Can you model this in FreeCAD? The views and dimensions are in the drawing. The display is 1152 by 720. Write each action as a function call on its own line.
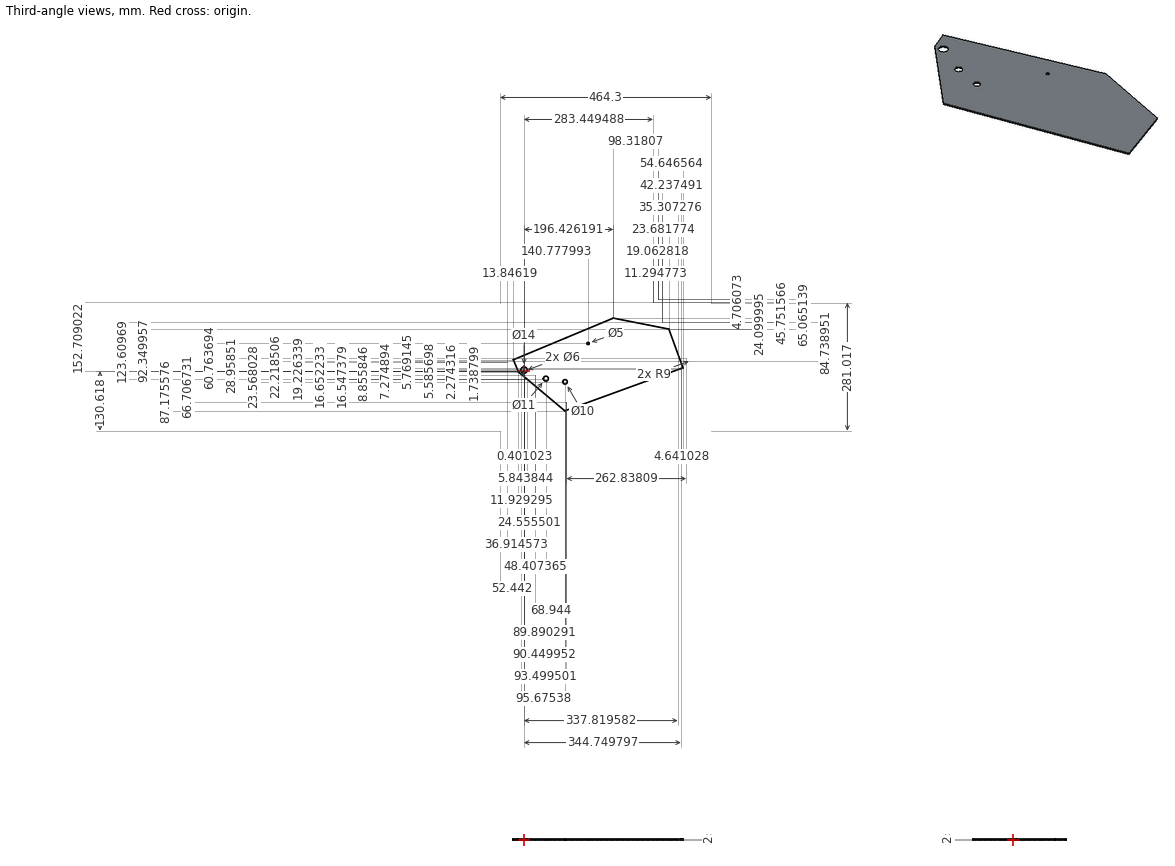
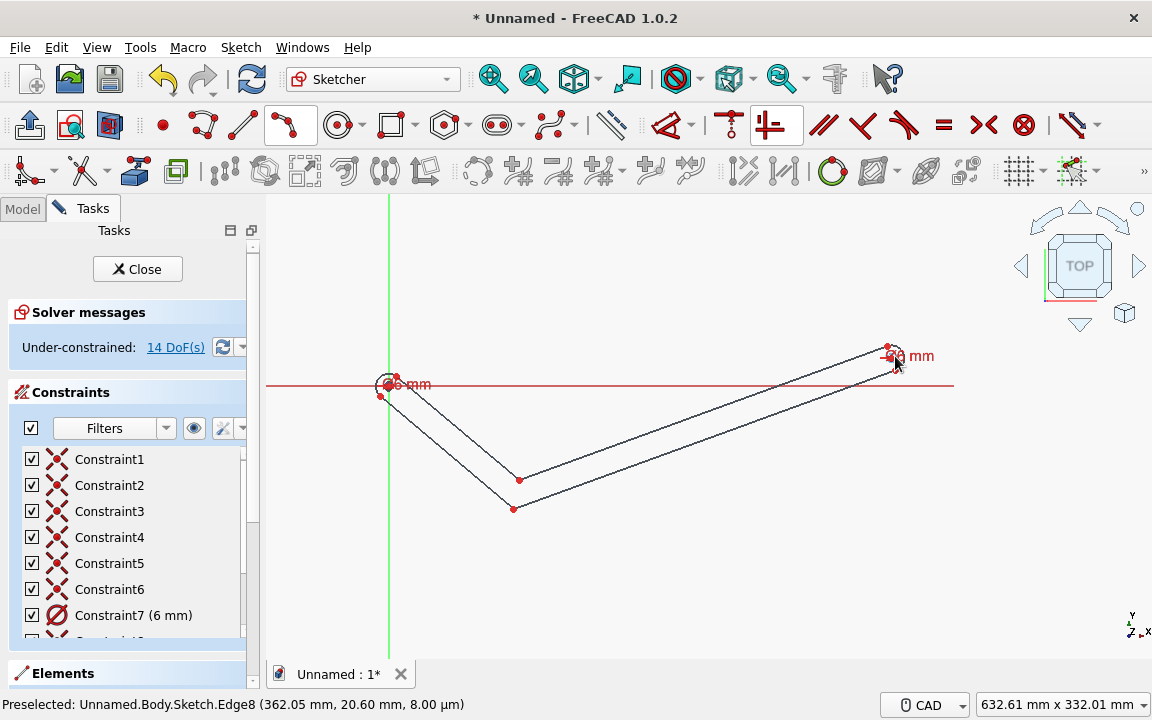
click(777, 386)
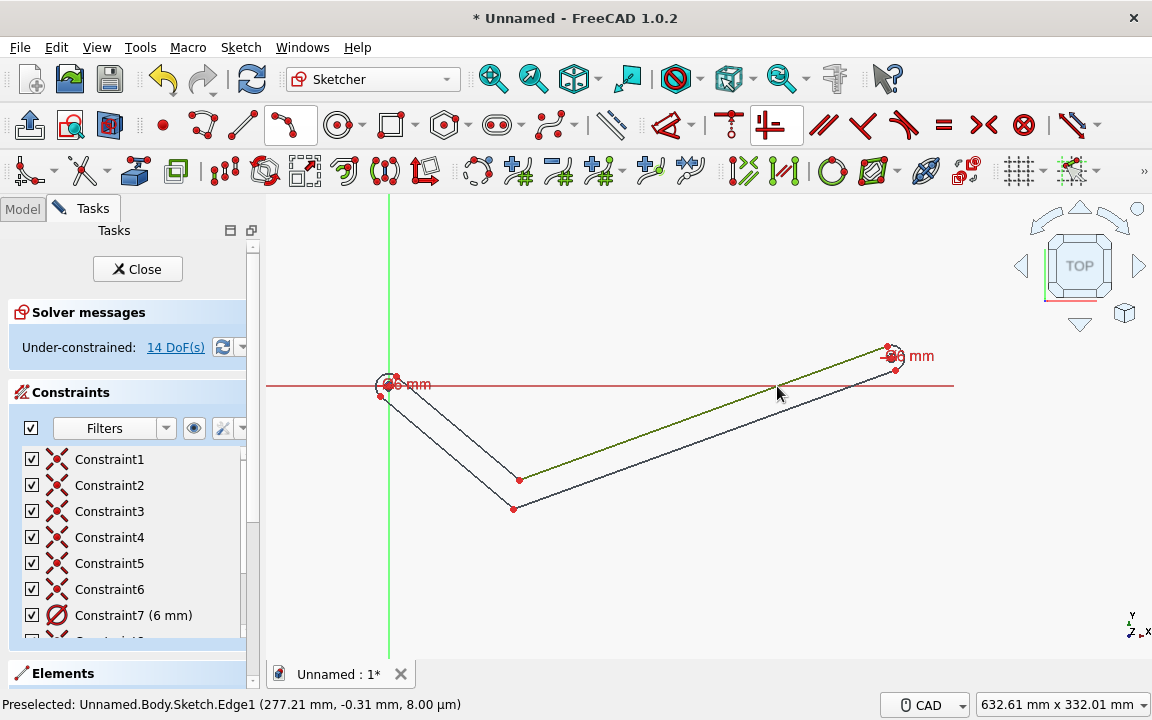
scroll(904, 354, up, 3)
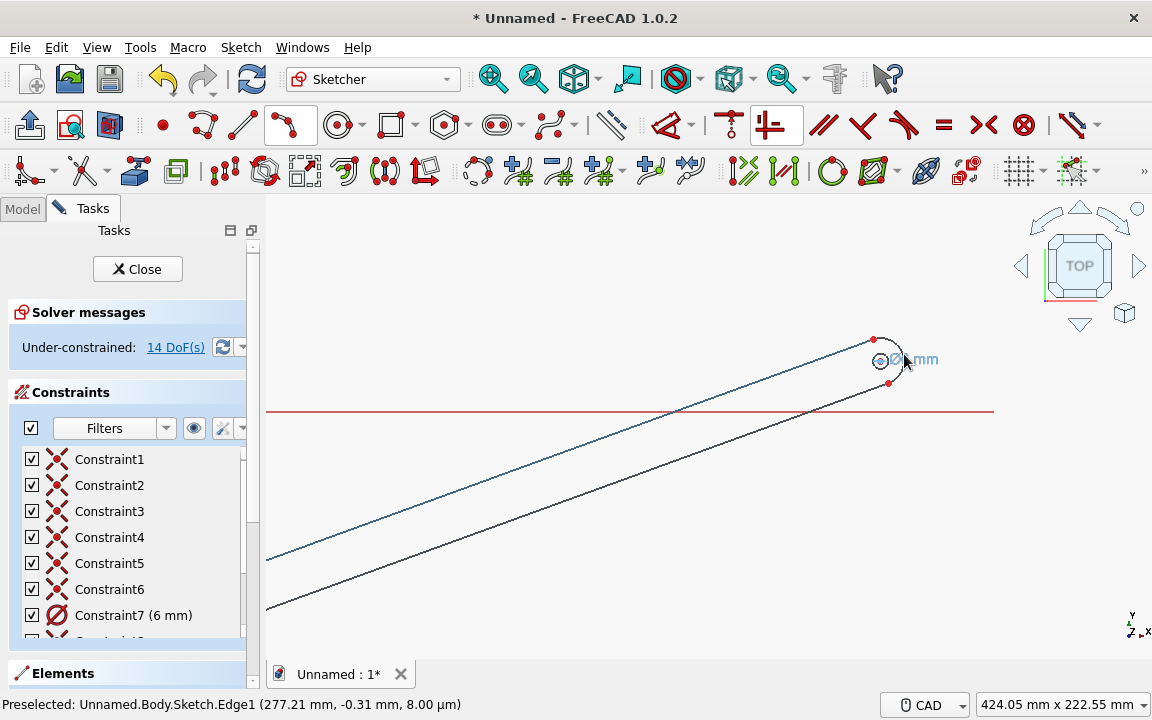
click(894, 342)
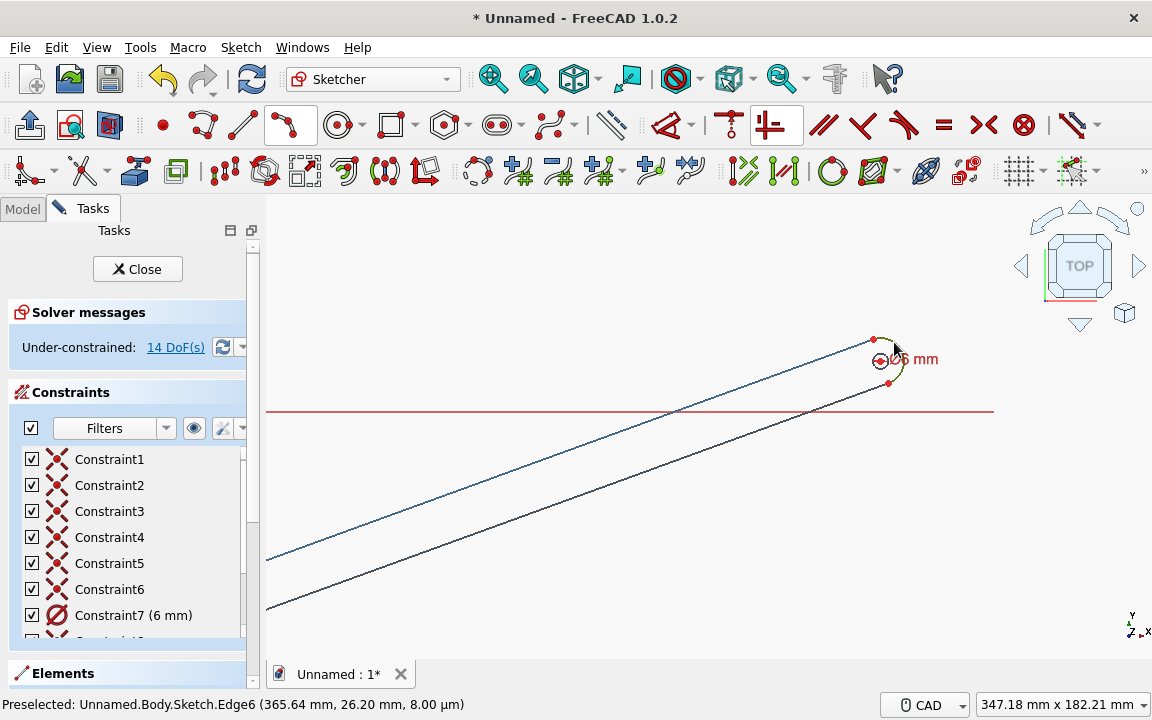
key(t)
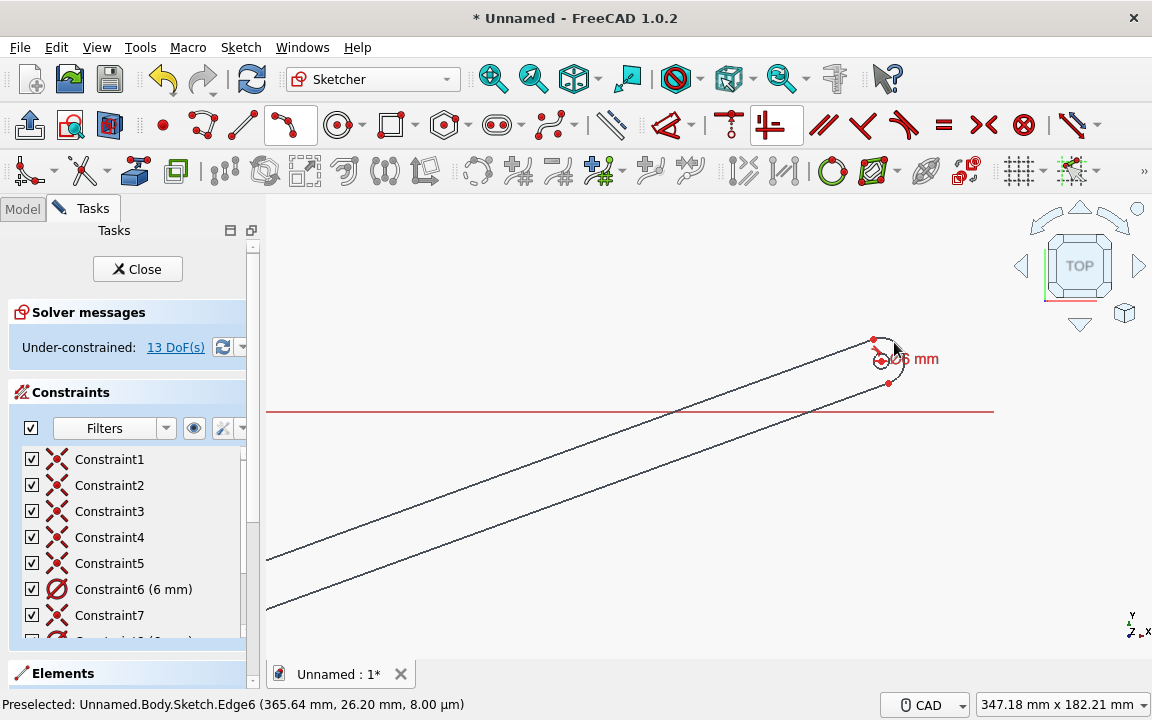
scroll(903, 354, down, 3)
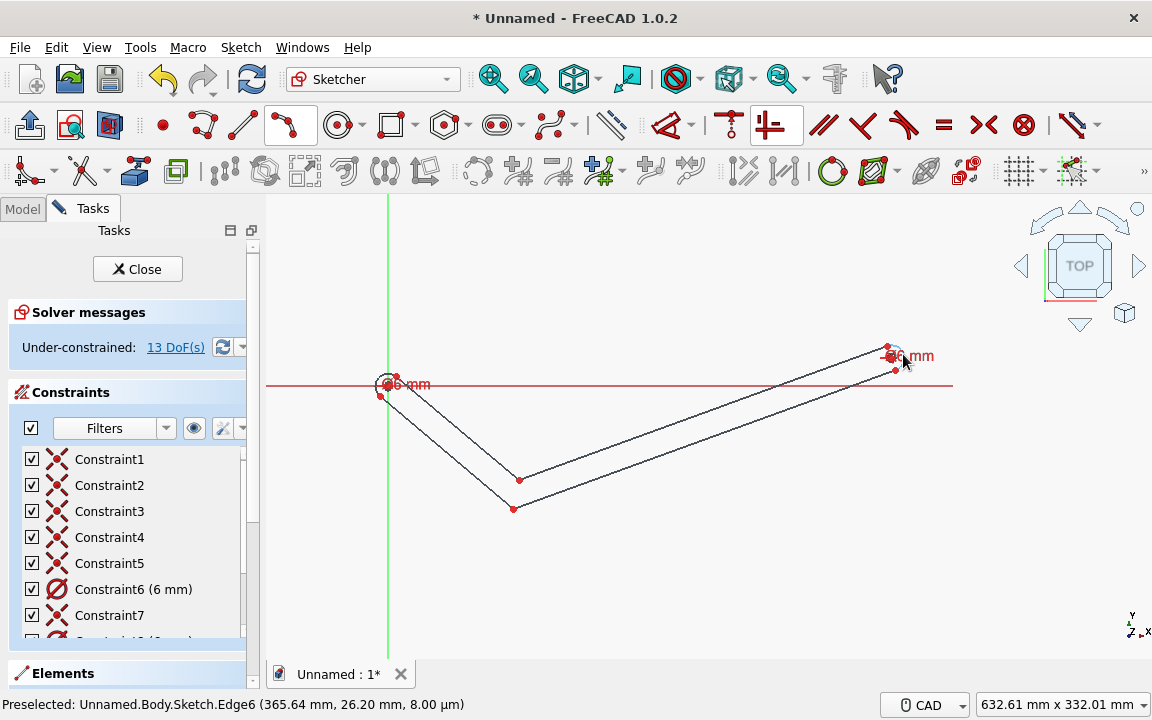
click(482, 449)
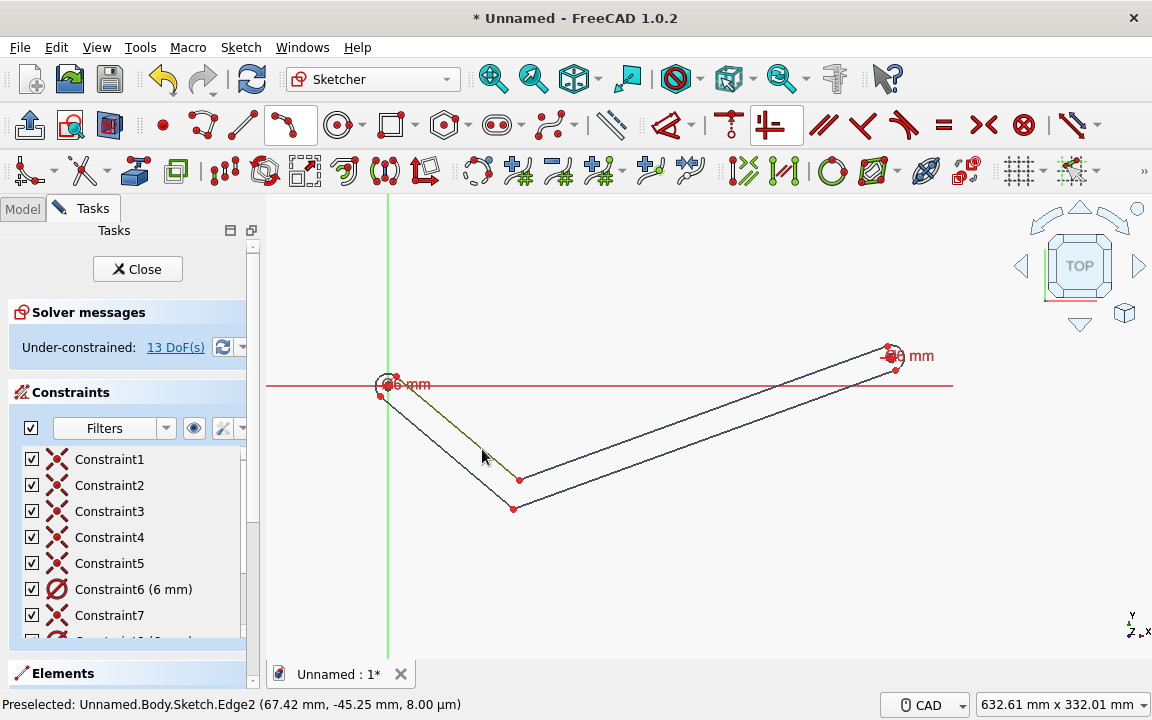
scroll(376, 386, up, 3)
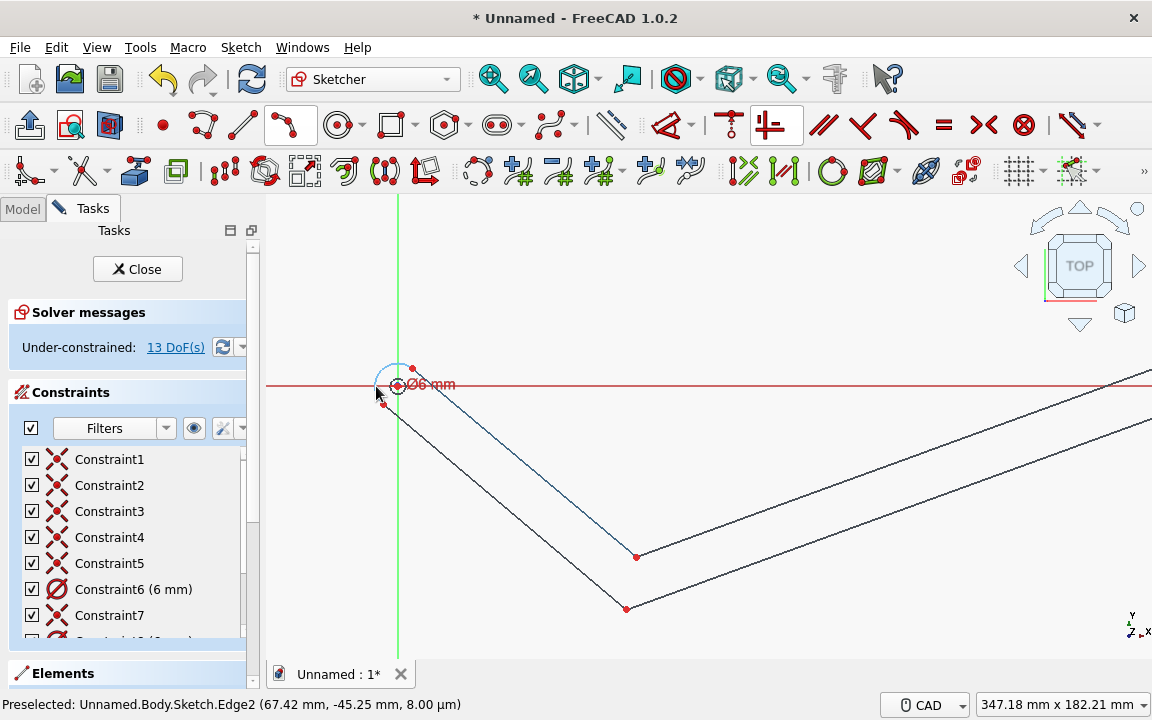
click(375, 385)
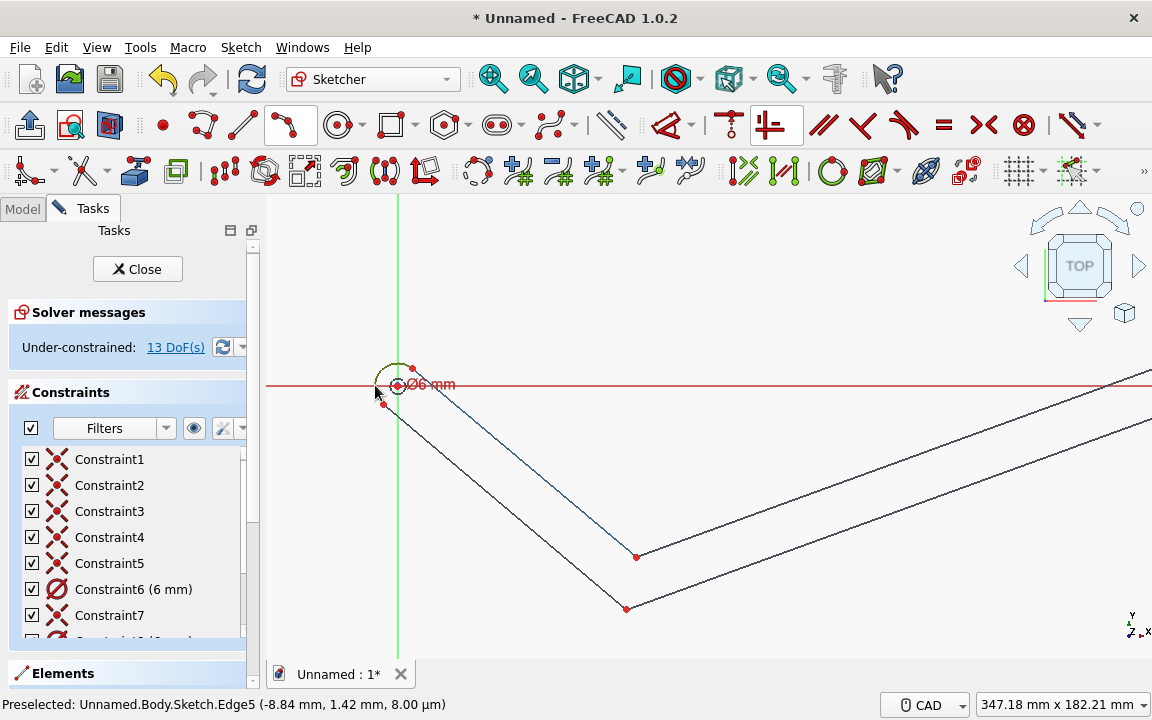
key(t)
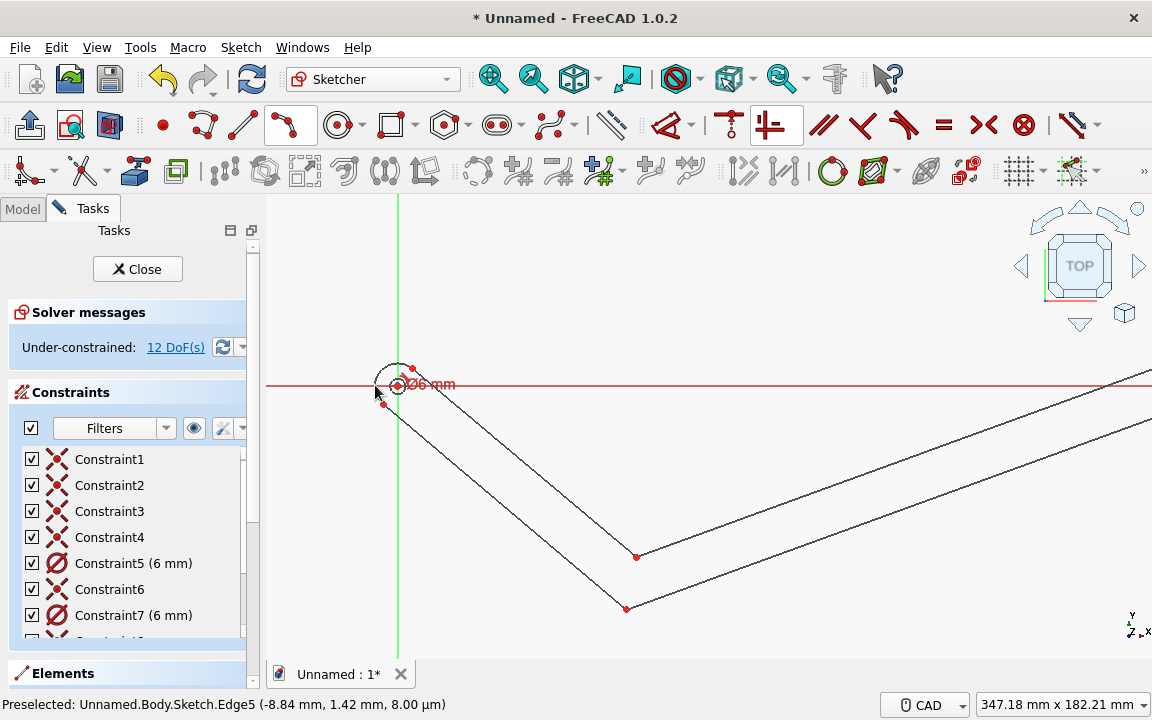
click(456, 466)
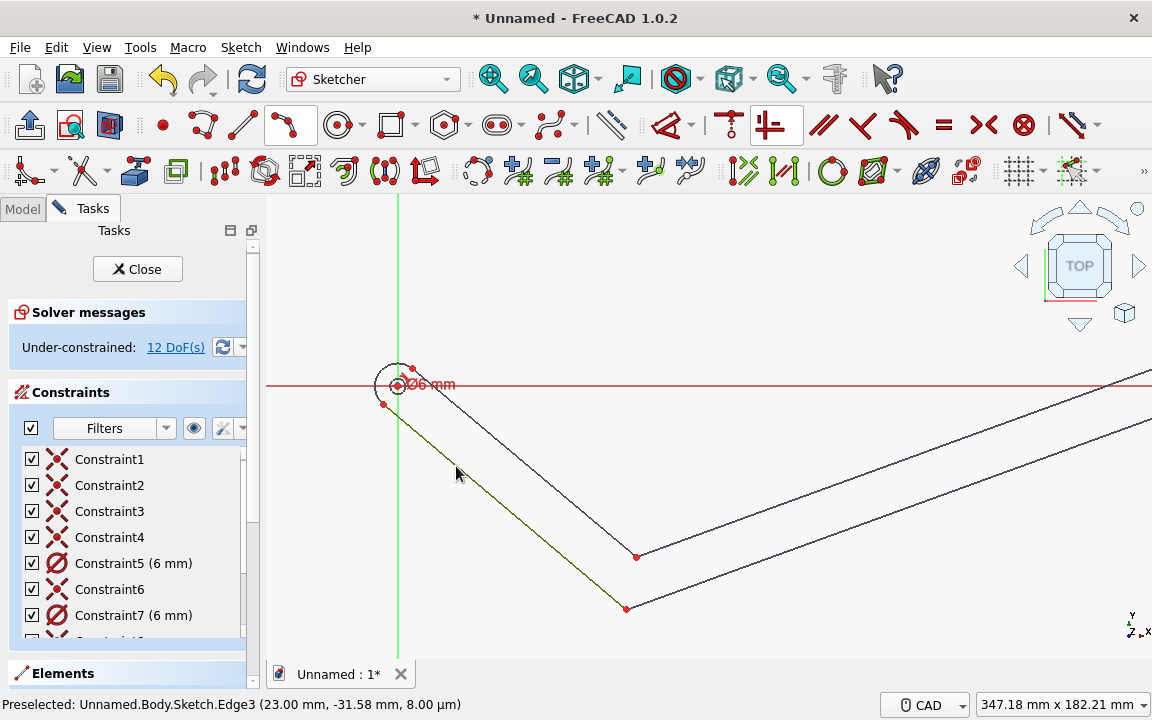
click(375, 385)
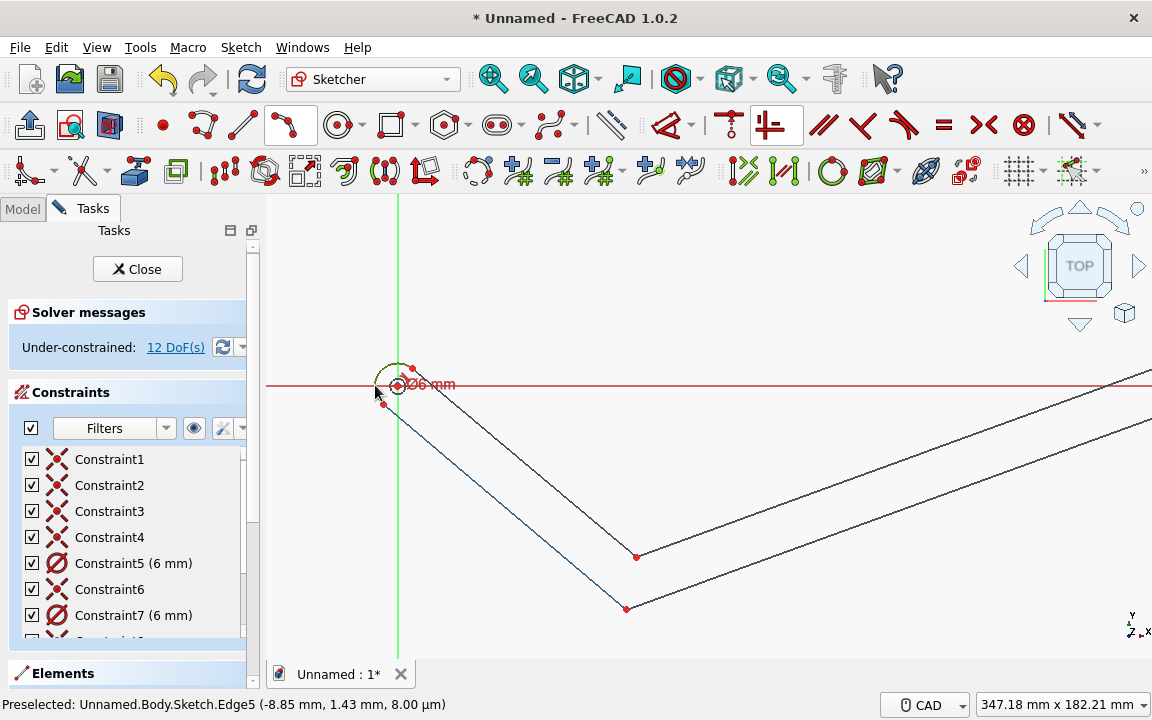
key(t)